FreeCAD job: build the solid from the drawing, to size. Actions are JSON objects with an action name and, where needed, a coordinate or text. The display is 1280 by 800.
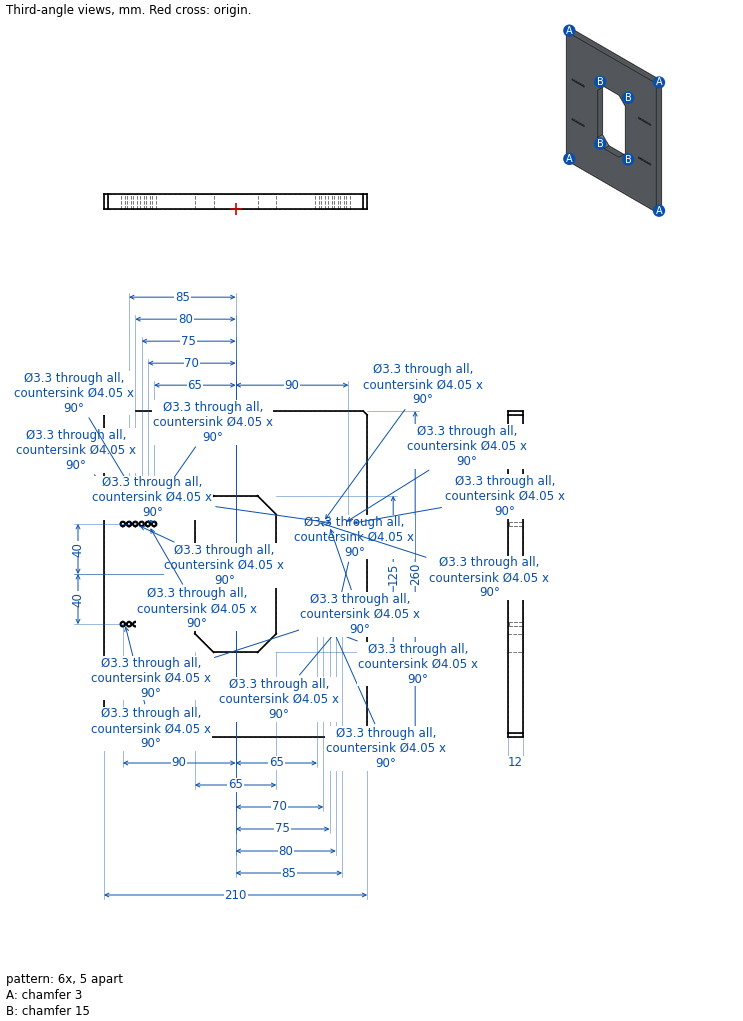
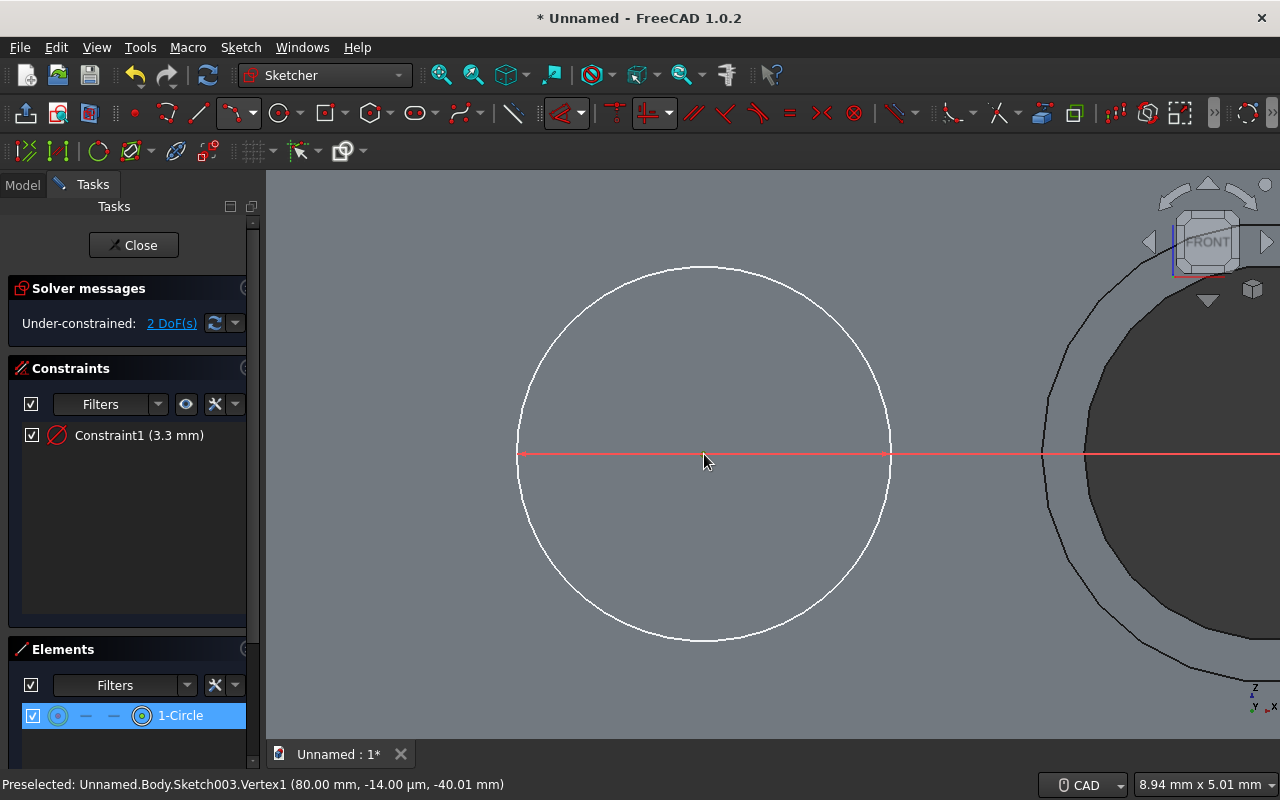
{"action": "key", "text": "l"}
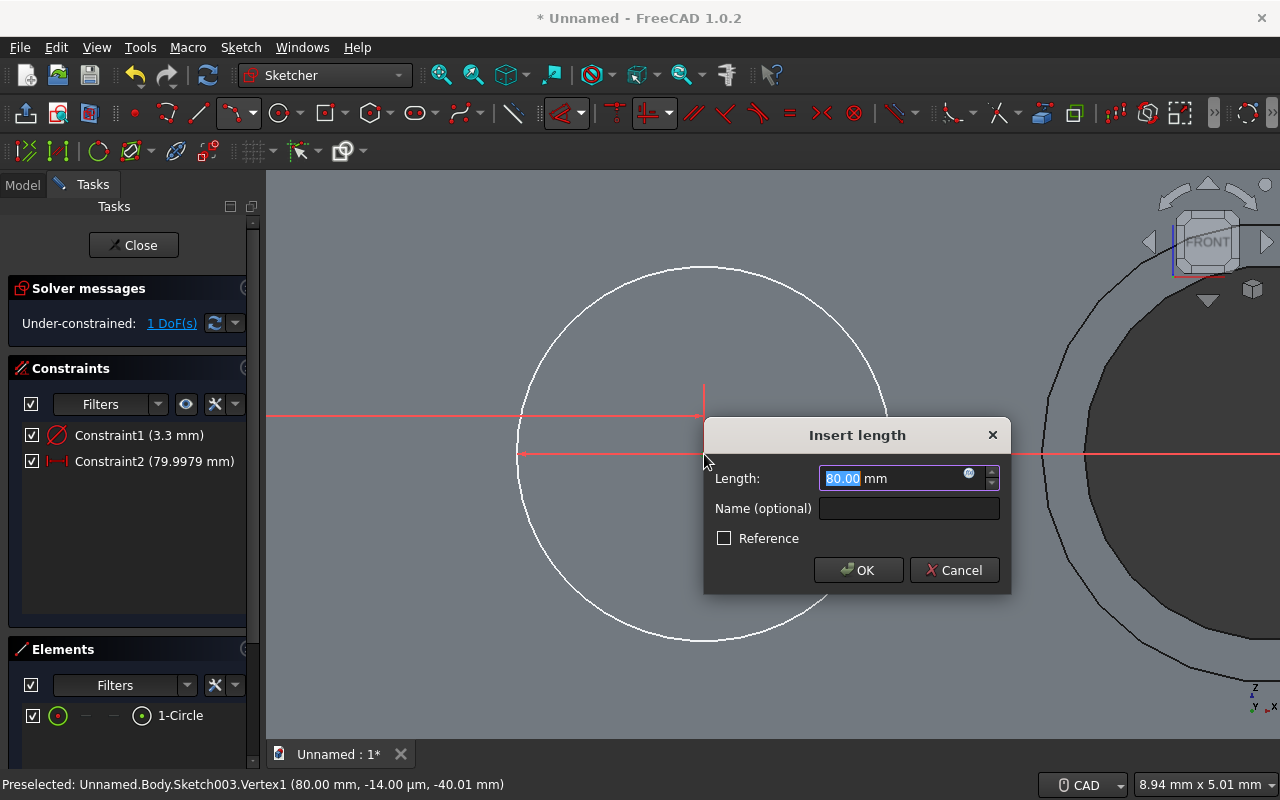
{"action": "type", "text": "80"}
{"action": "key", "text": "Return"}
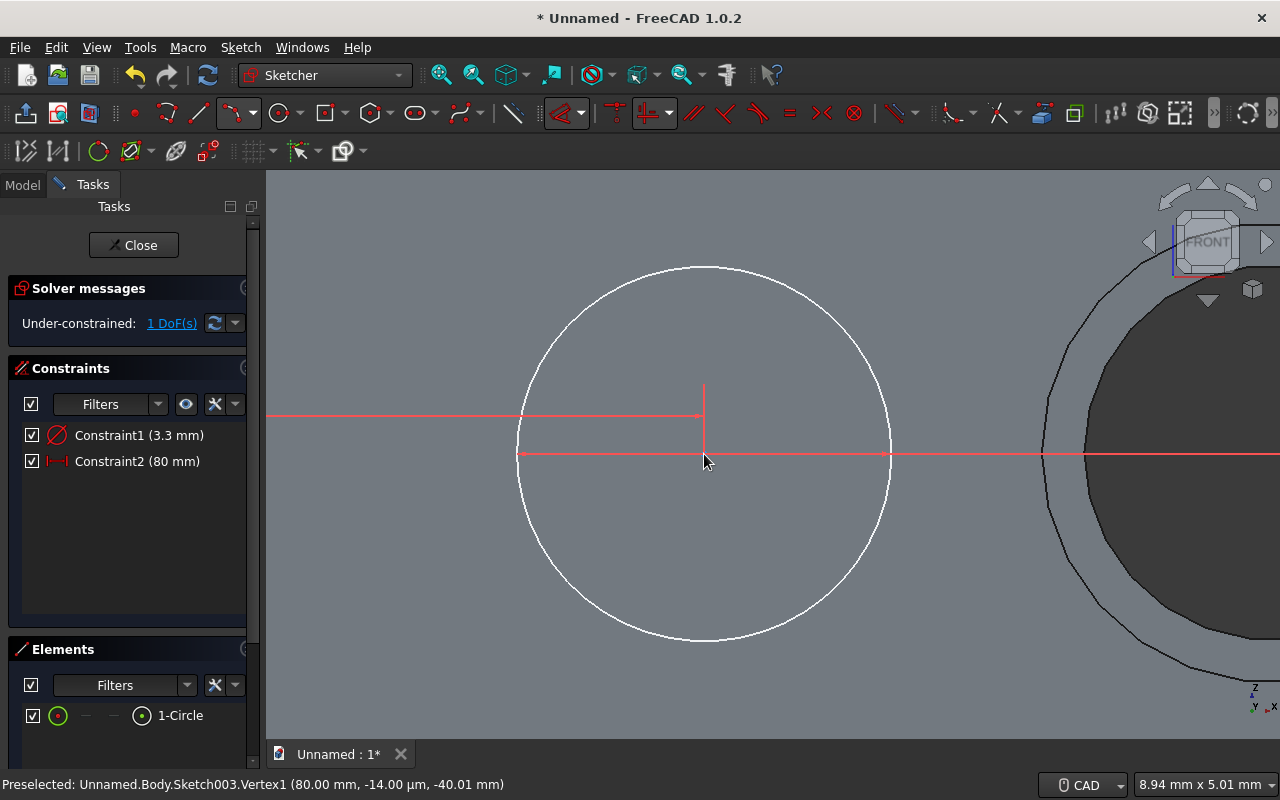
{"action": "left_click", "coordinate": [704, 454]}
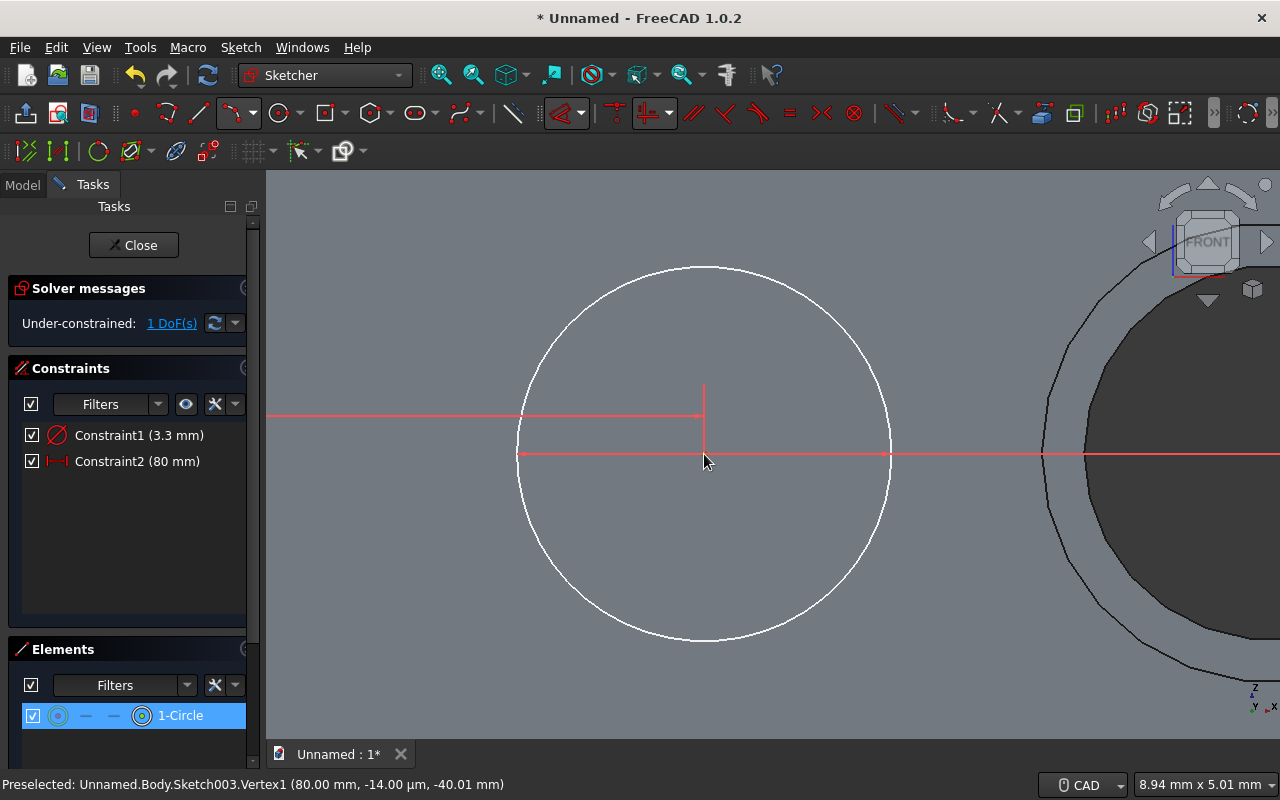
{"action": "left_click", "coordinate": [584, 114]}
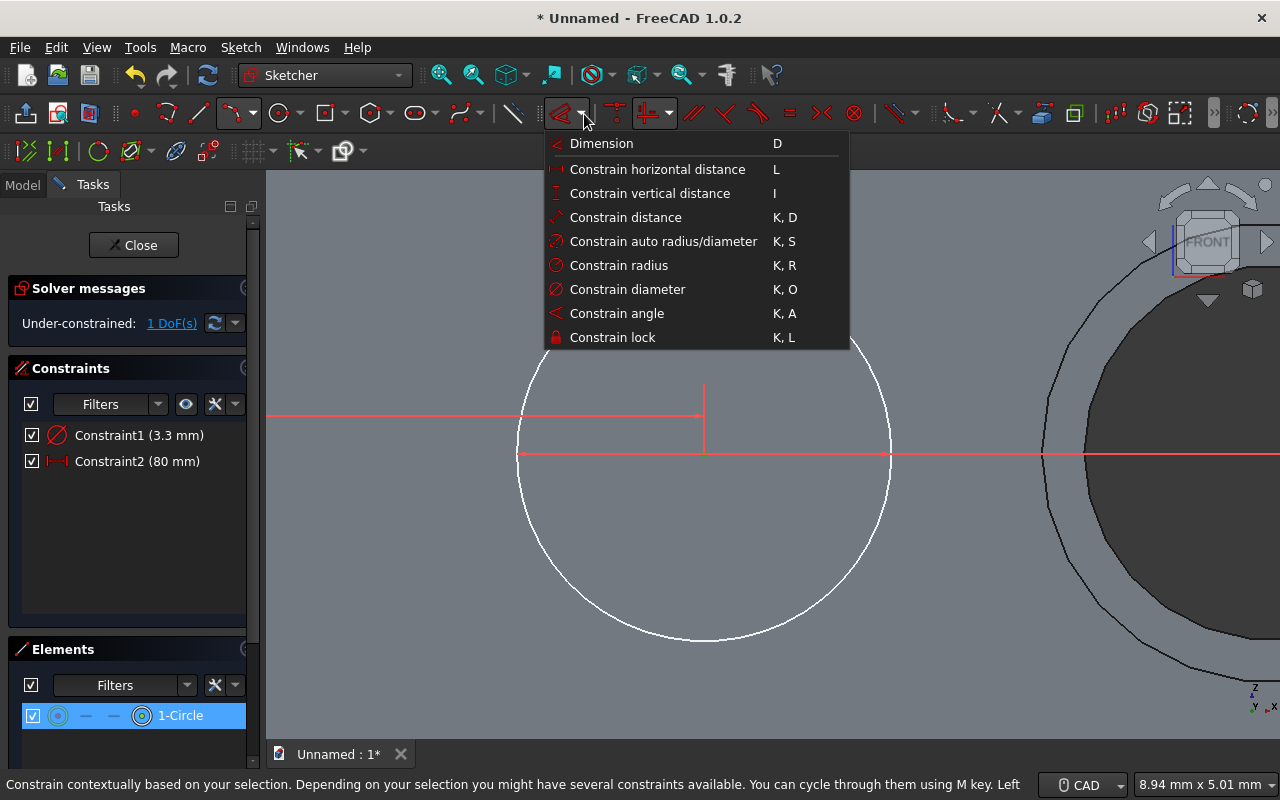
{"action": "left_click", "coordinate": [697, 193]}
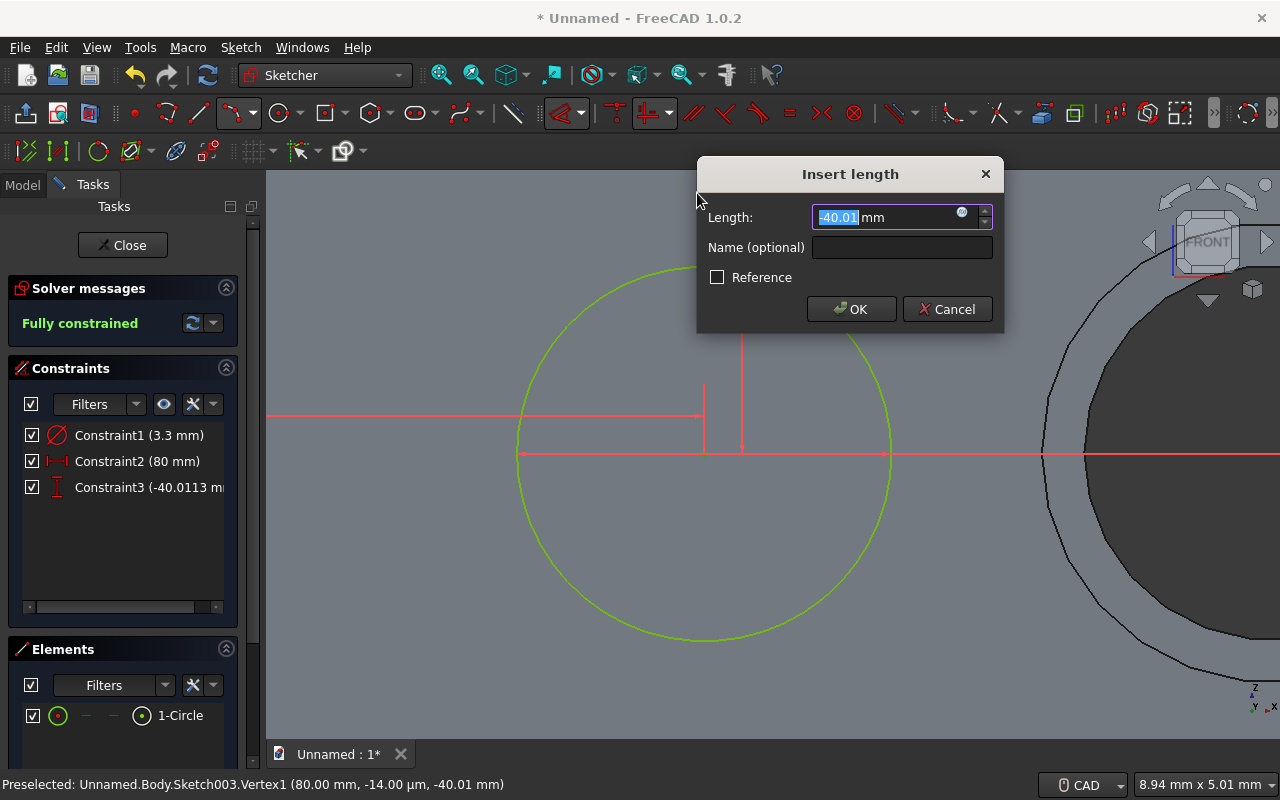
{"action": "type", "text": "-40"}
{"action": "key", "text": "Return"}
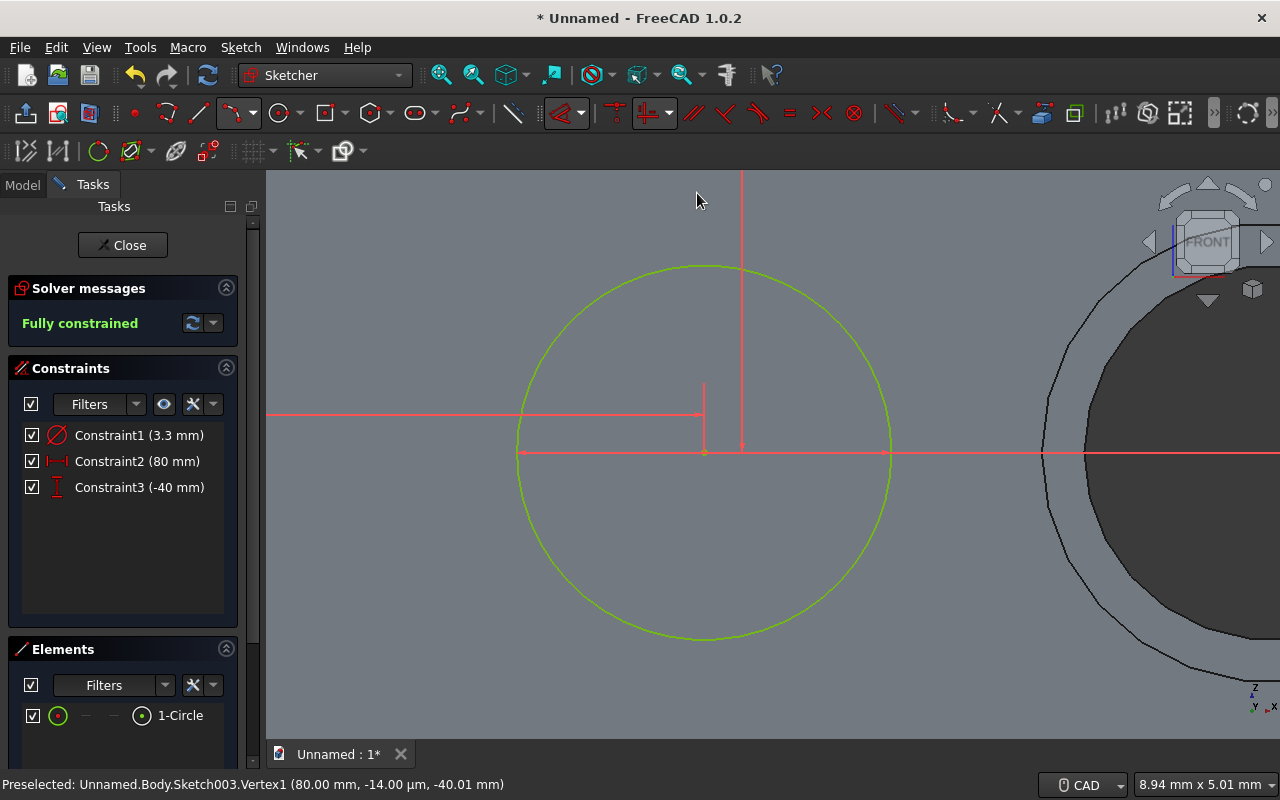
{"action": "left_click", "coordinate": [123, 245]}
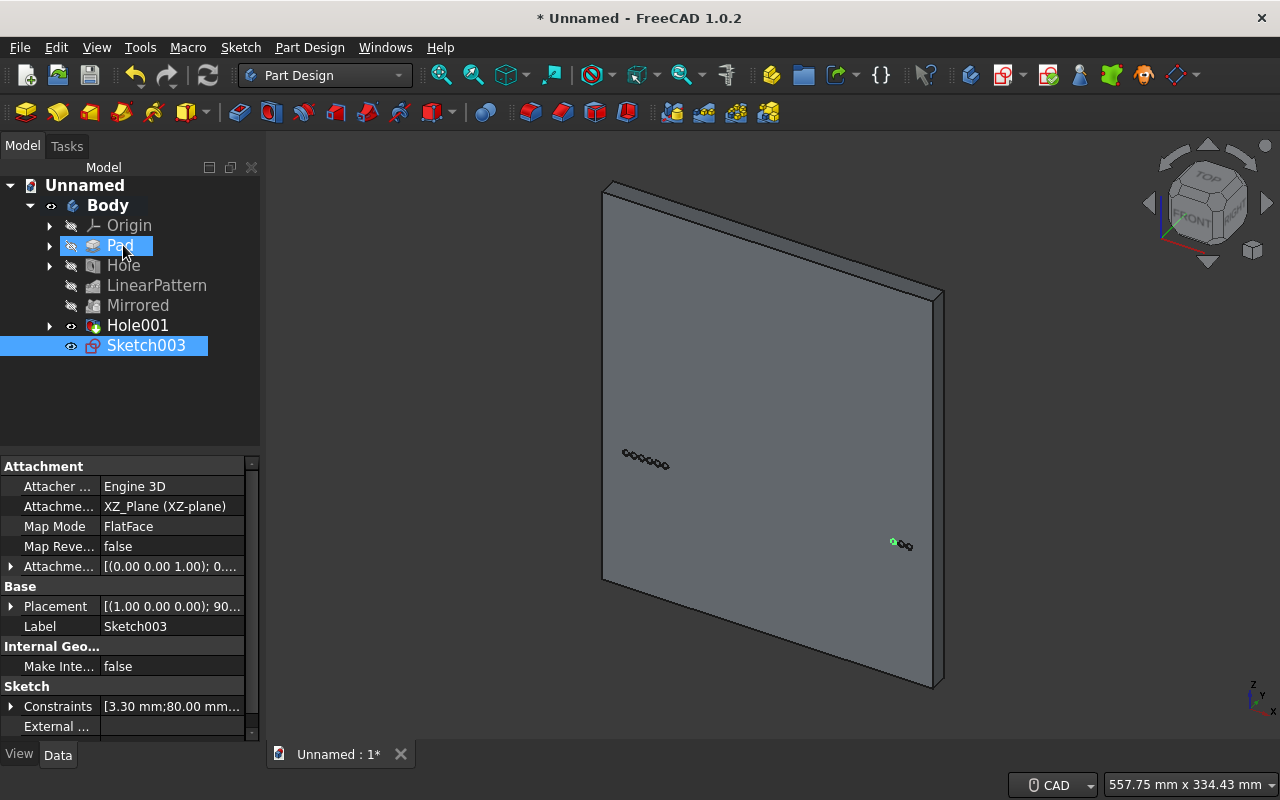
{"action": "left_click", "coordinate": [272, 112]}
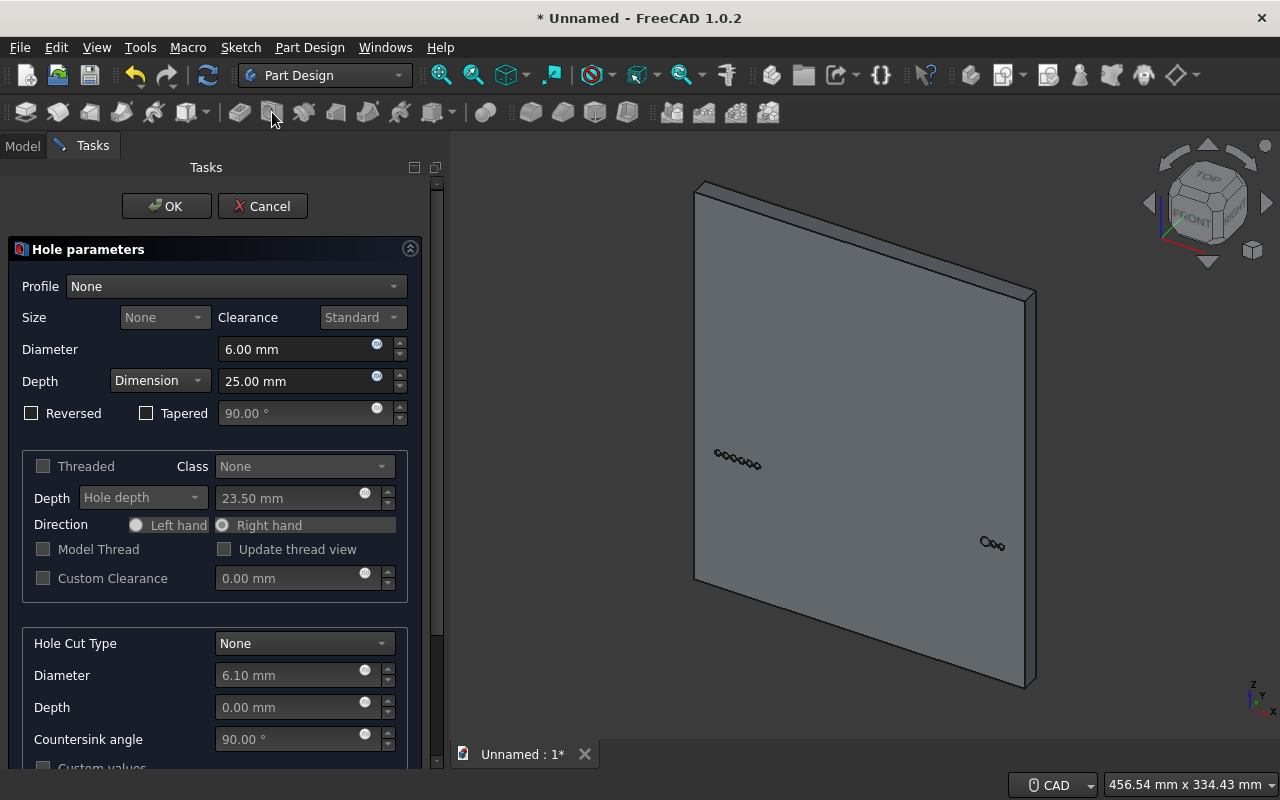
{"action": "triple_click", "coordinate": [305, 349]}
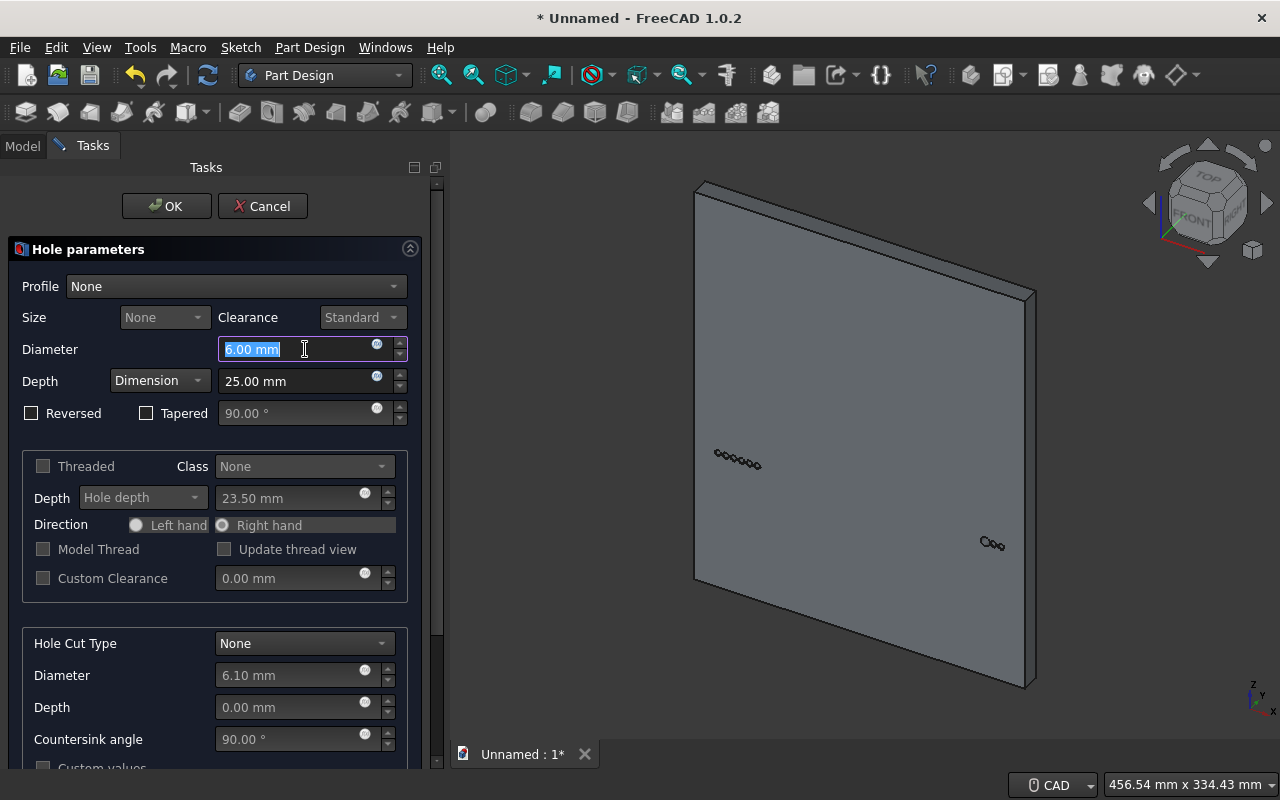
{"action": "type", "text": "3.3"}
{"action": "key", "text": "Tab"}